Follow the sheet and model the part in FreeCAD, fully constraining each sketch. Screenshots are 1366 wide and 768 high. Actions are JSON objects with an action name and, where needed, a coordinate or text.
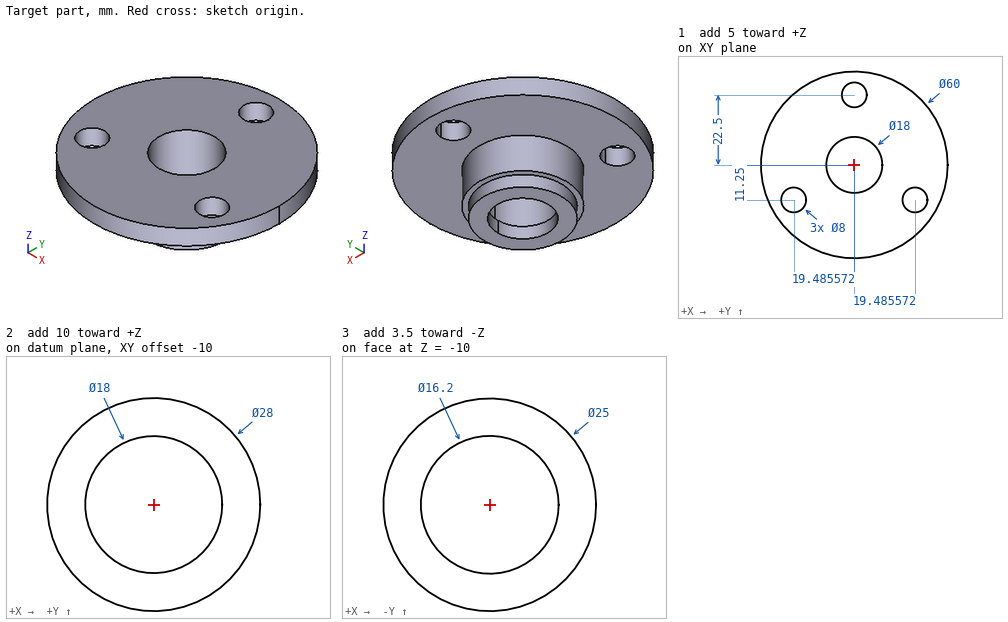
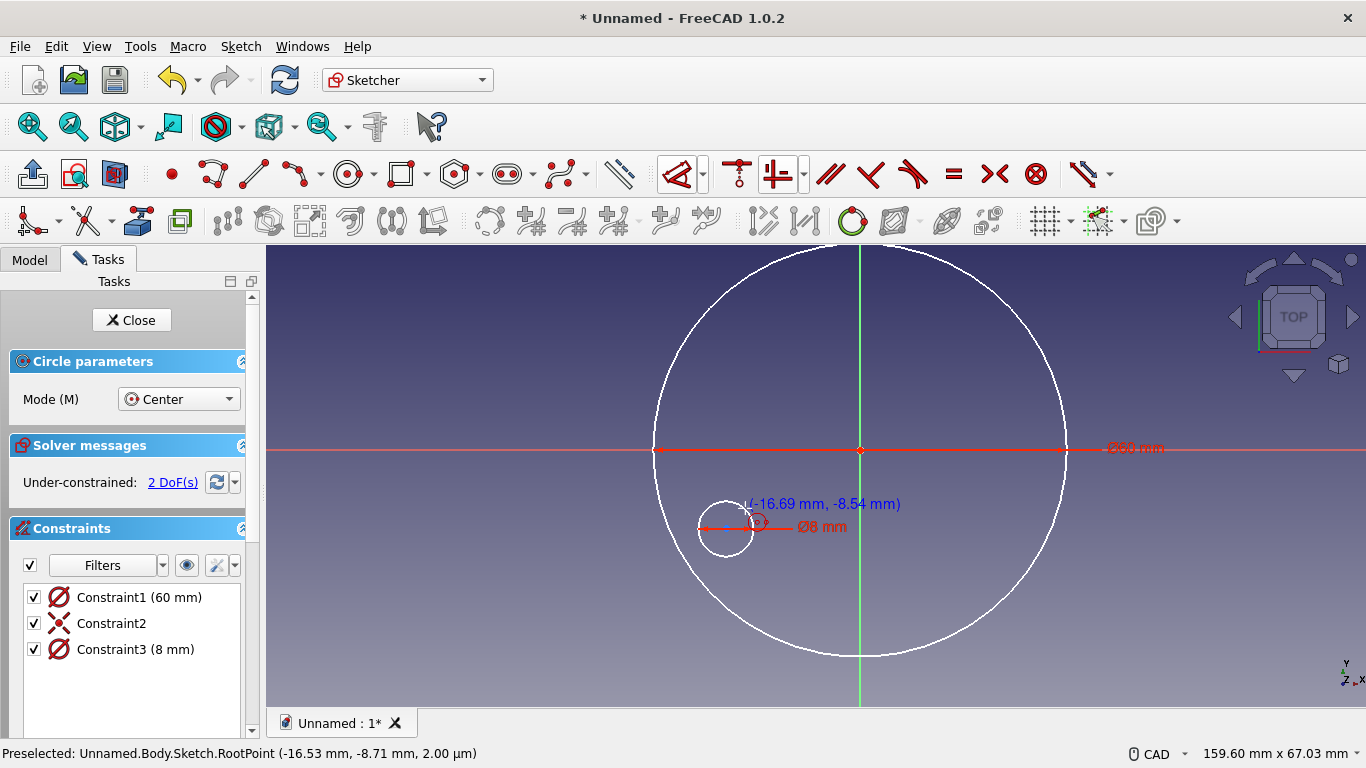
{"action": "left_click", "coordinate": [994, 528]}
{"action": "mouse_move", "coordinate": [1014, 508]}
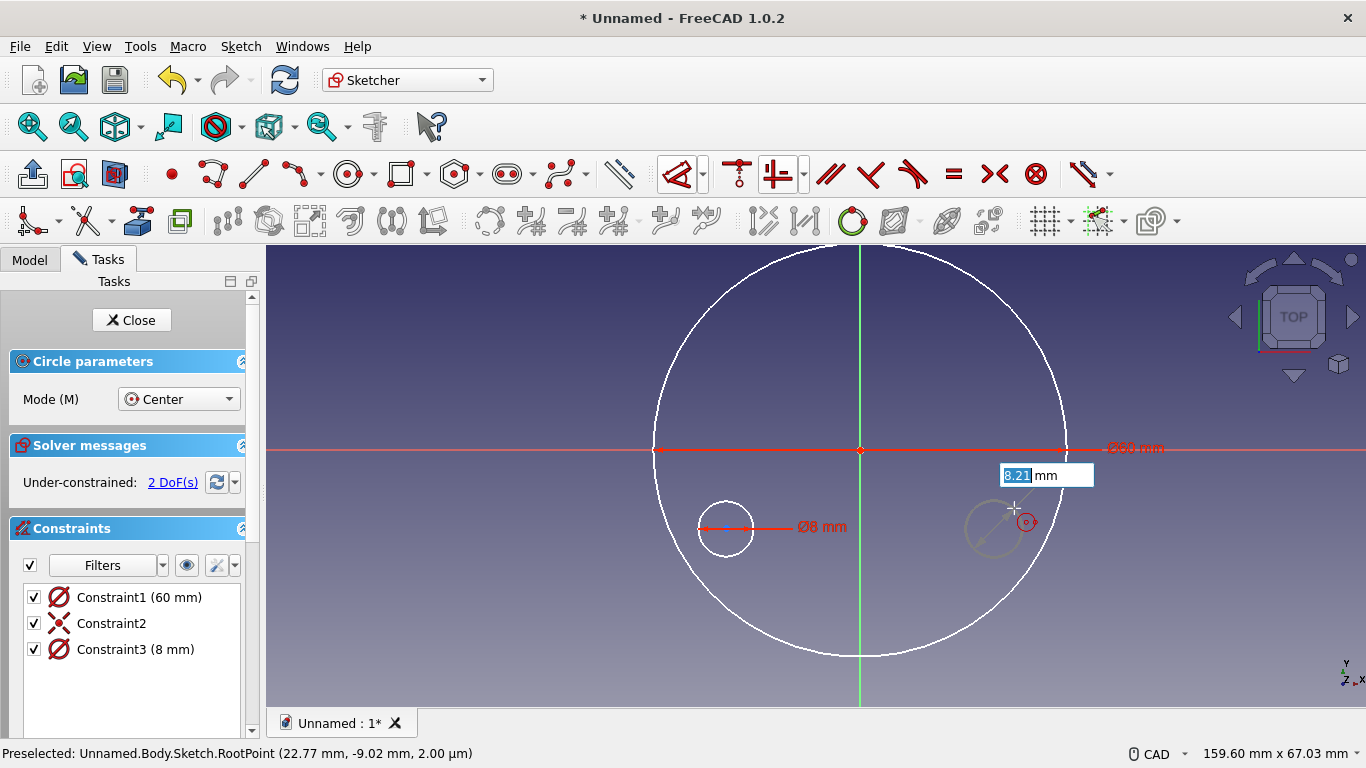
{"action": "type", "text": "8"}
{"action": "key", "text": "Return"}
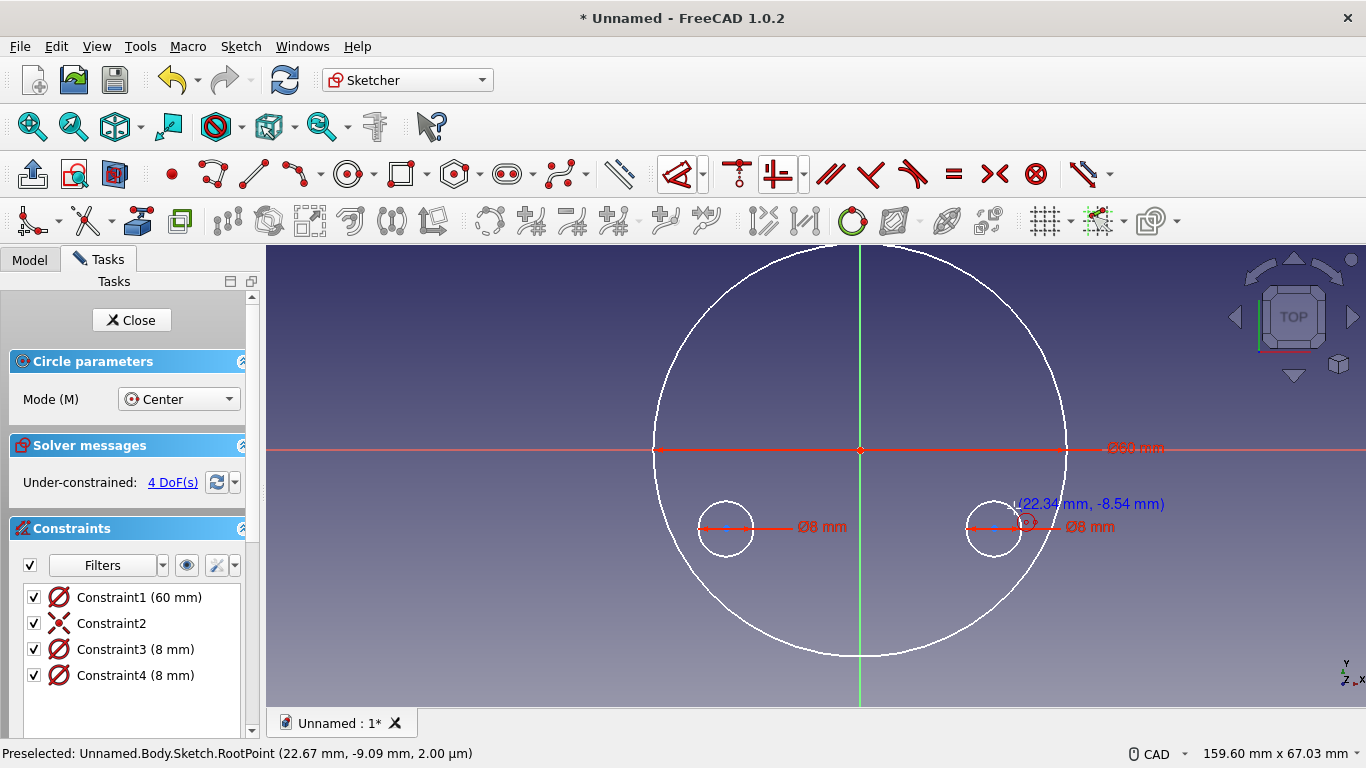
{"action": "left_click", "coordinate": [860, 450]}
{"action": "mouse_move", "coordinate": [904, 406]}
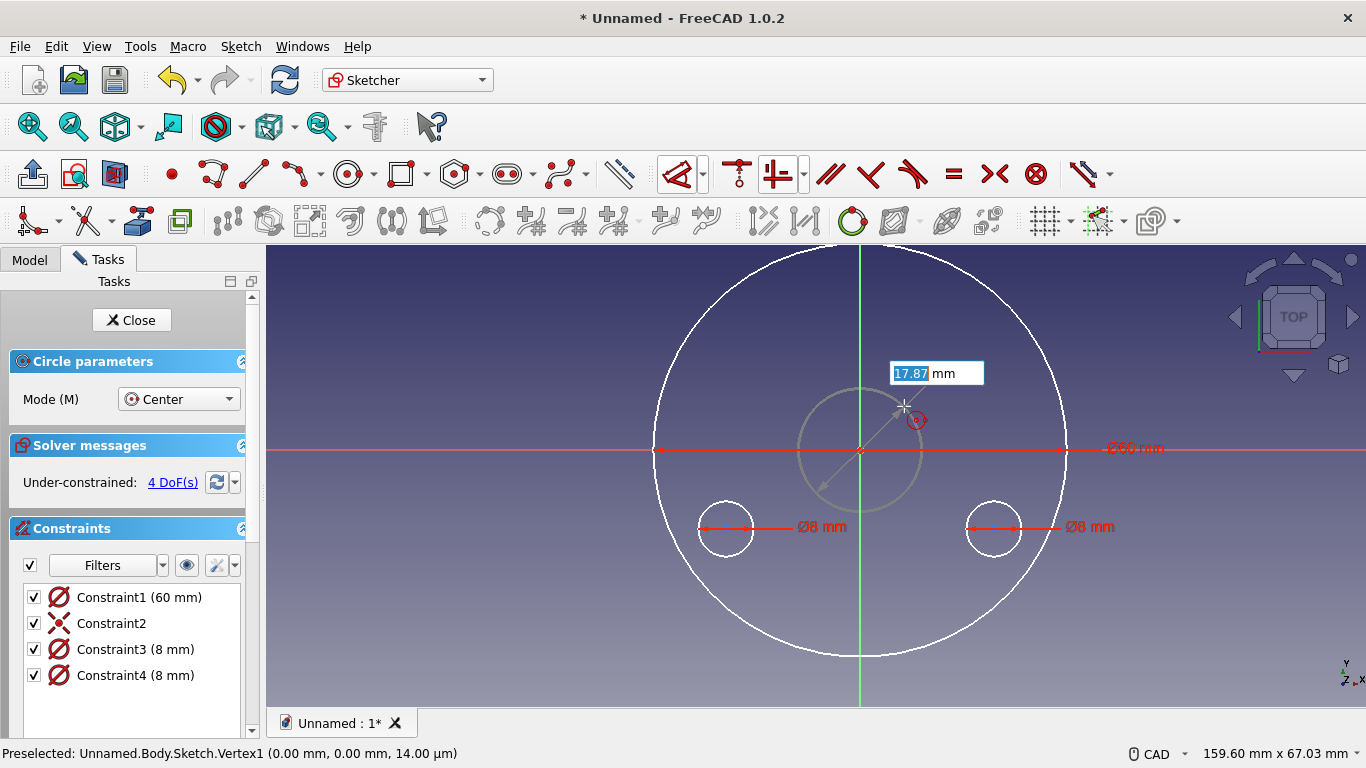
{"action": "type", "text": "18"}
{"action": "key", "text": "Return"}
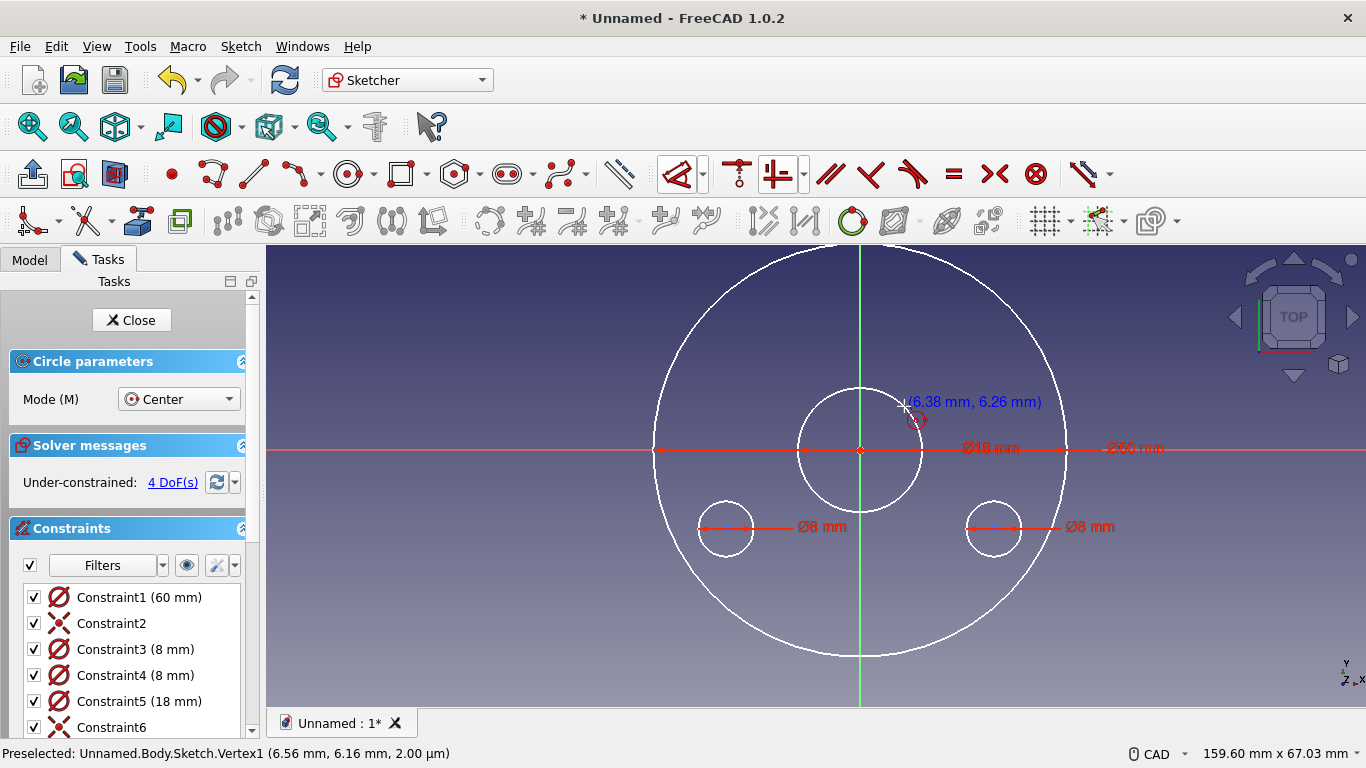
{"action": "left_click", "coordinate": [860, 295]}
{"action": "mouse_move", "coordinate": [880, 276]}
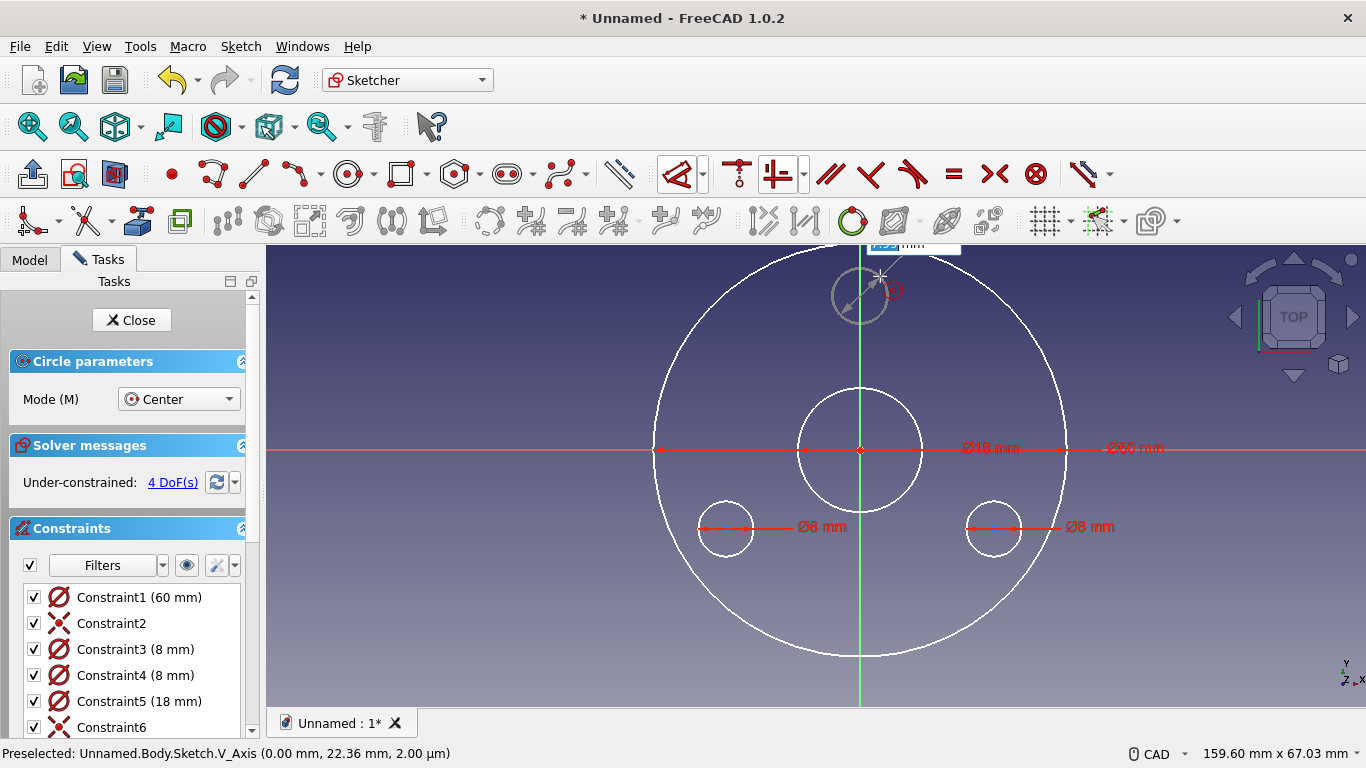
{"action": "type", "text": "8"}
{"action": "key", "text": "Return"}
{"action": "key", "text": "Escape"}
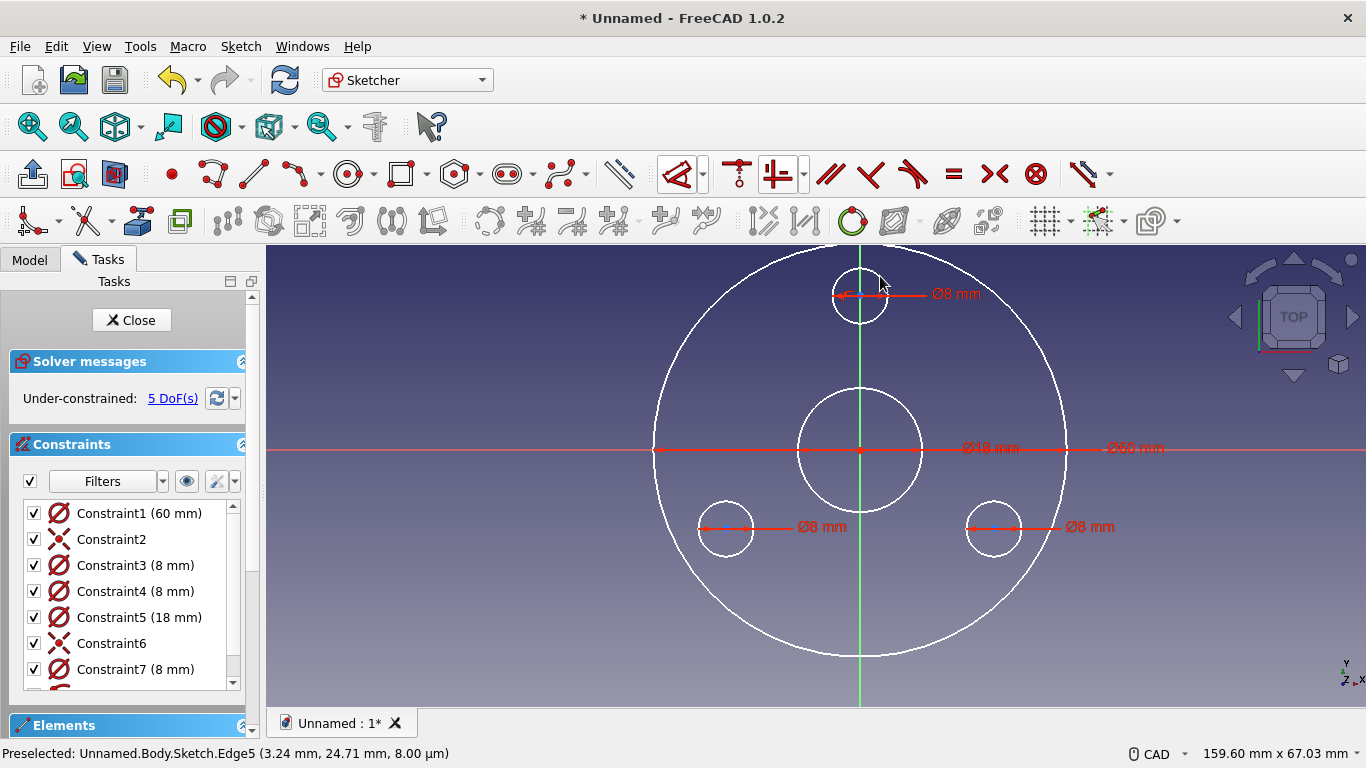
{"action": "left_click", "coordinate": [726, 529]}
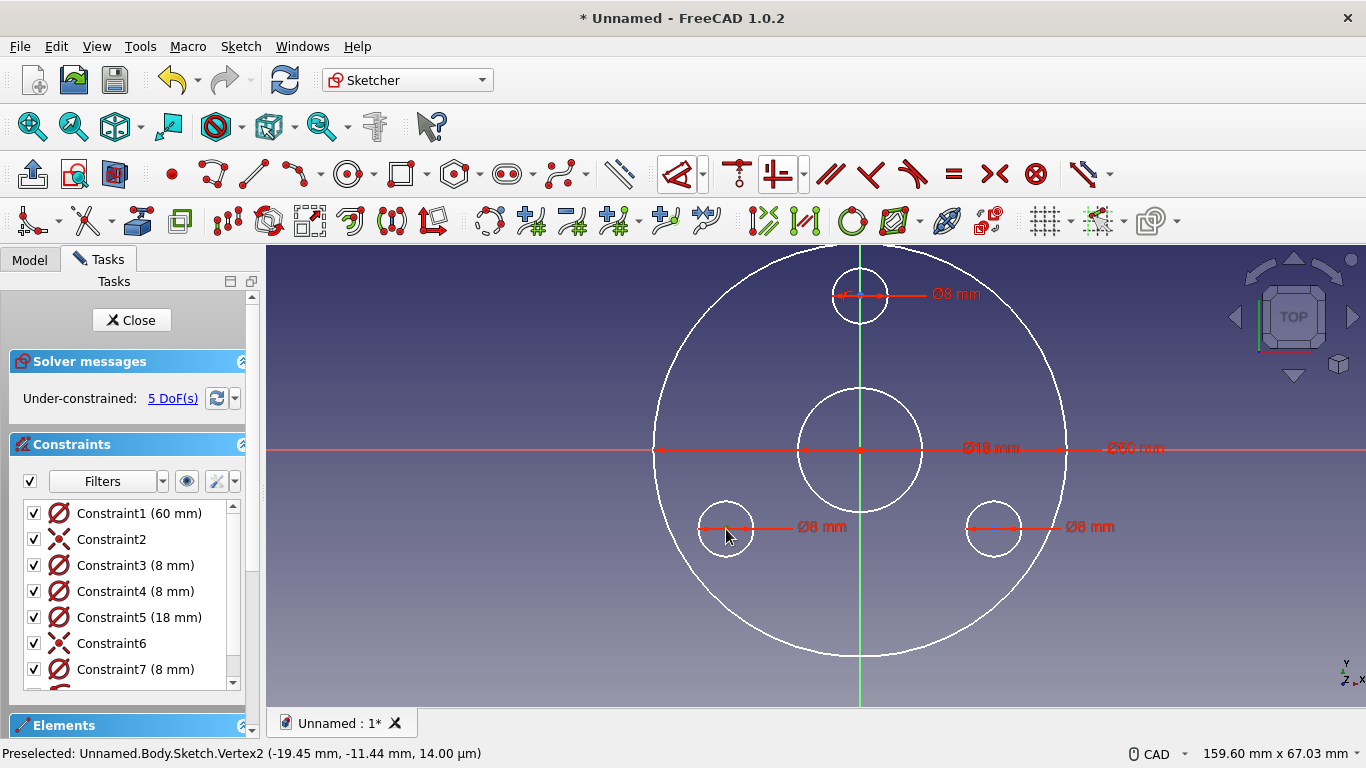
{"action": "left_click", "coordinate": [994, 529]}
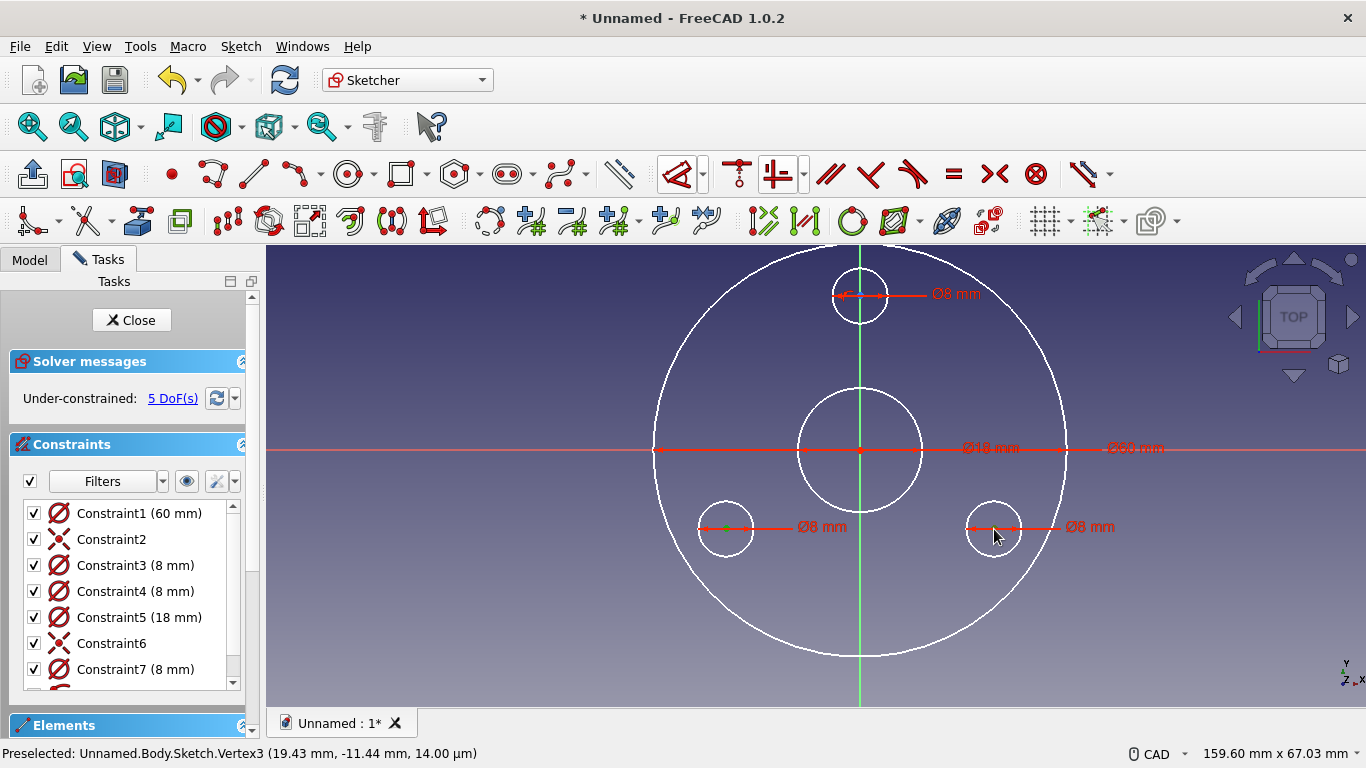
{"action": "left_click", "coordinate": [804, 174]}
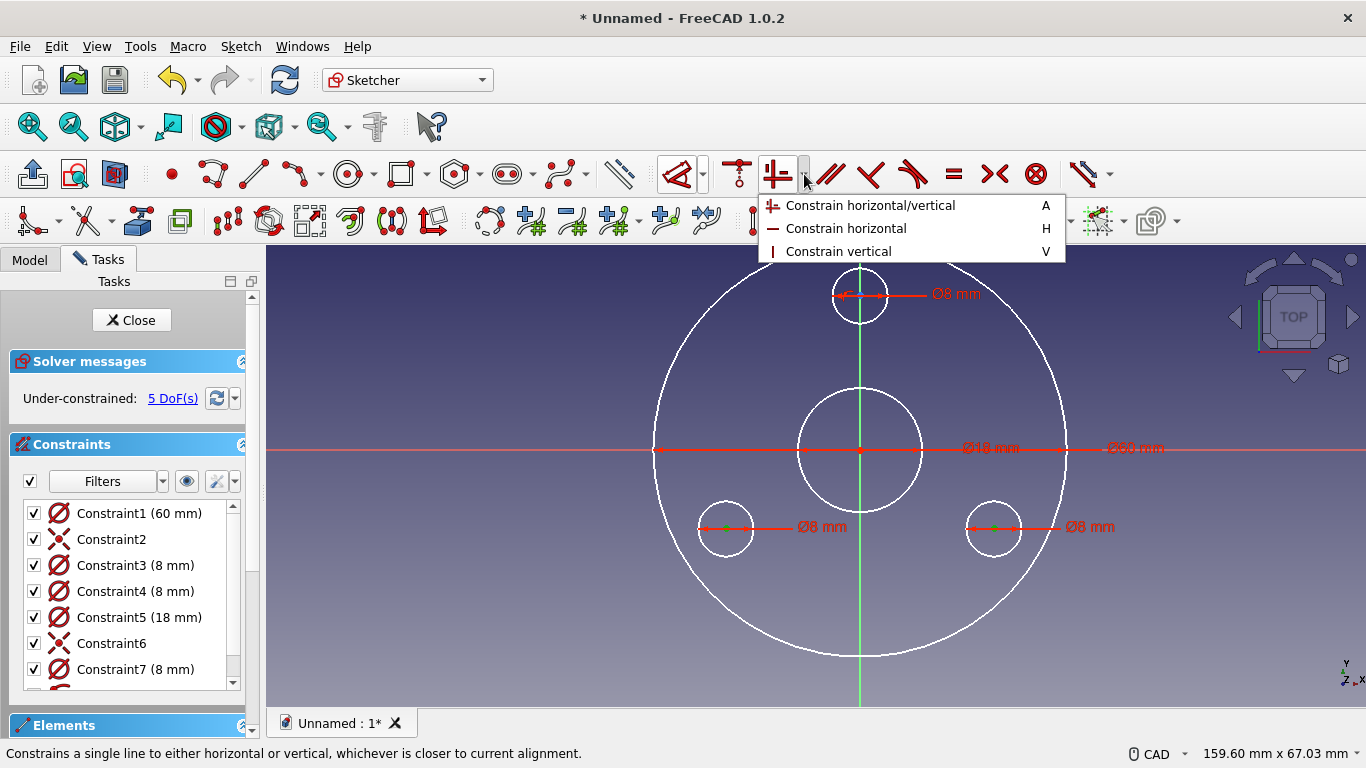
{"action": "left_click", "coordinate": [912, 228]}